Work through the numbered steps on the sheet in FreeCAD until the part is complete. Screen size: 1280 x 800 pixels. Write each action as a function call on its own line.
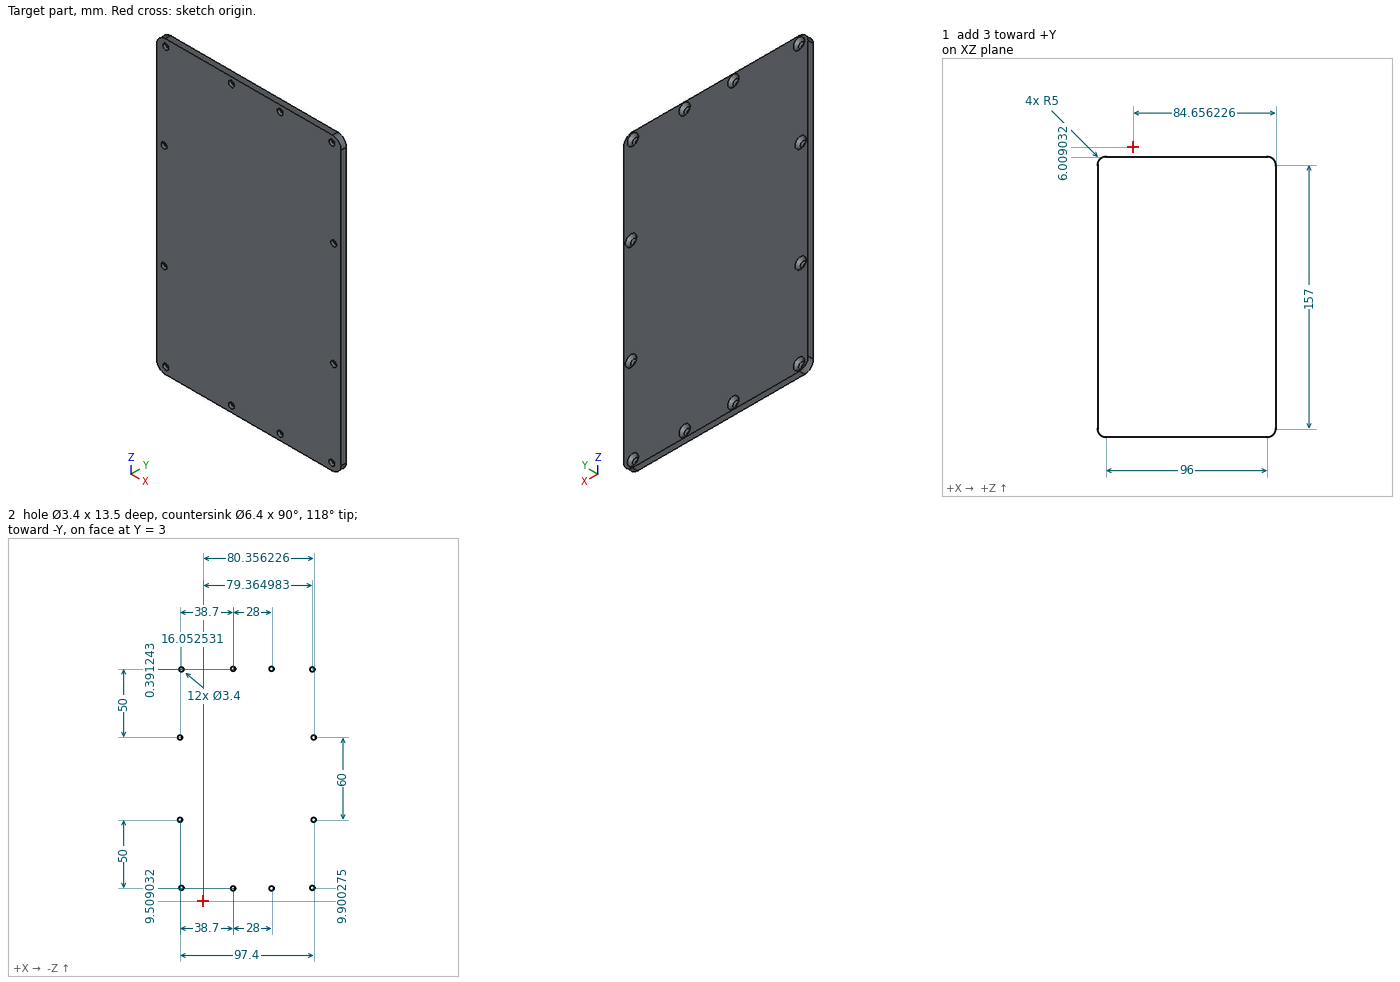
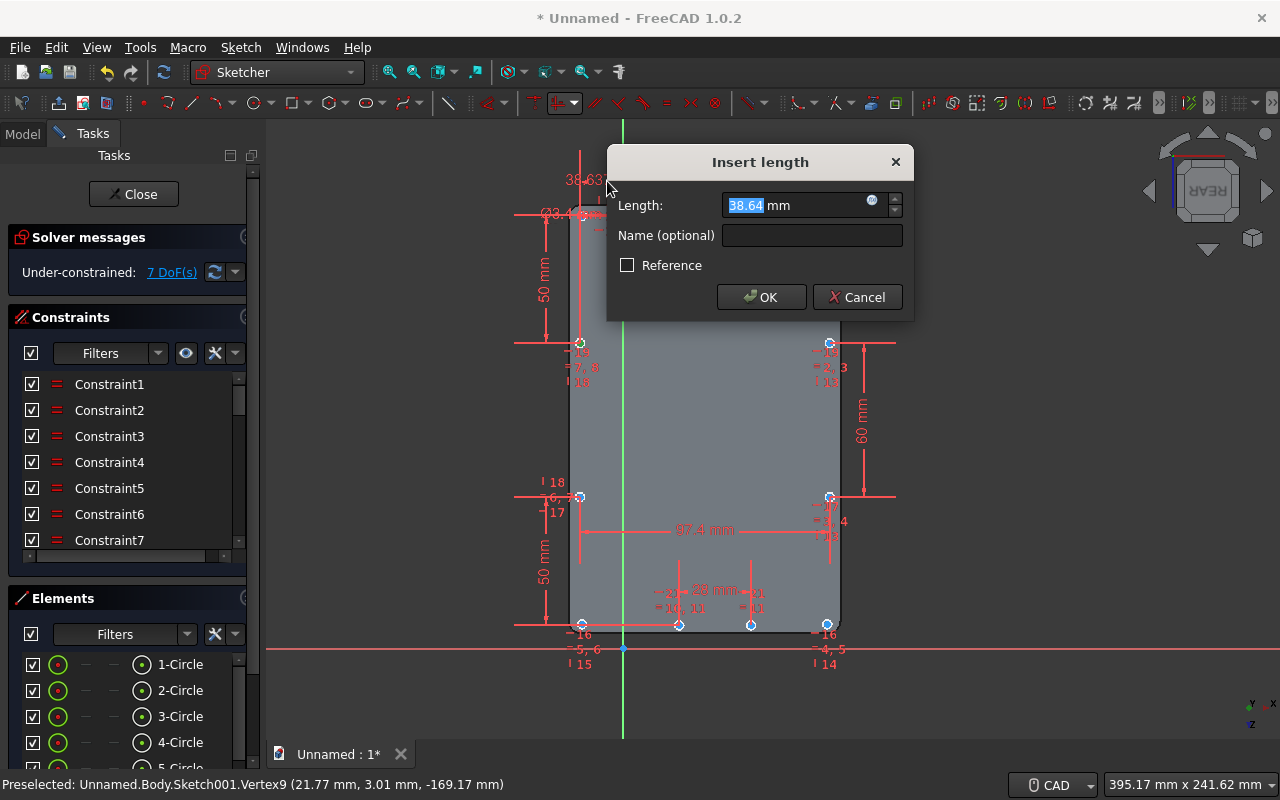
text(38.7)
key(Return)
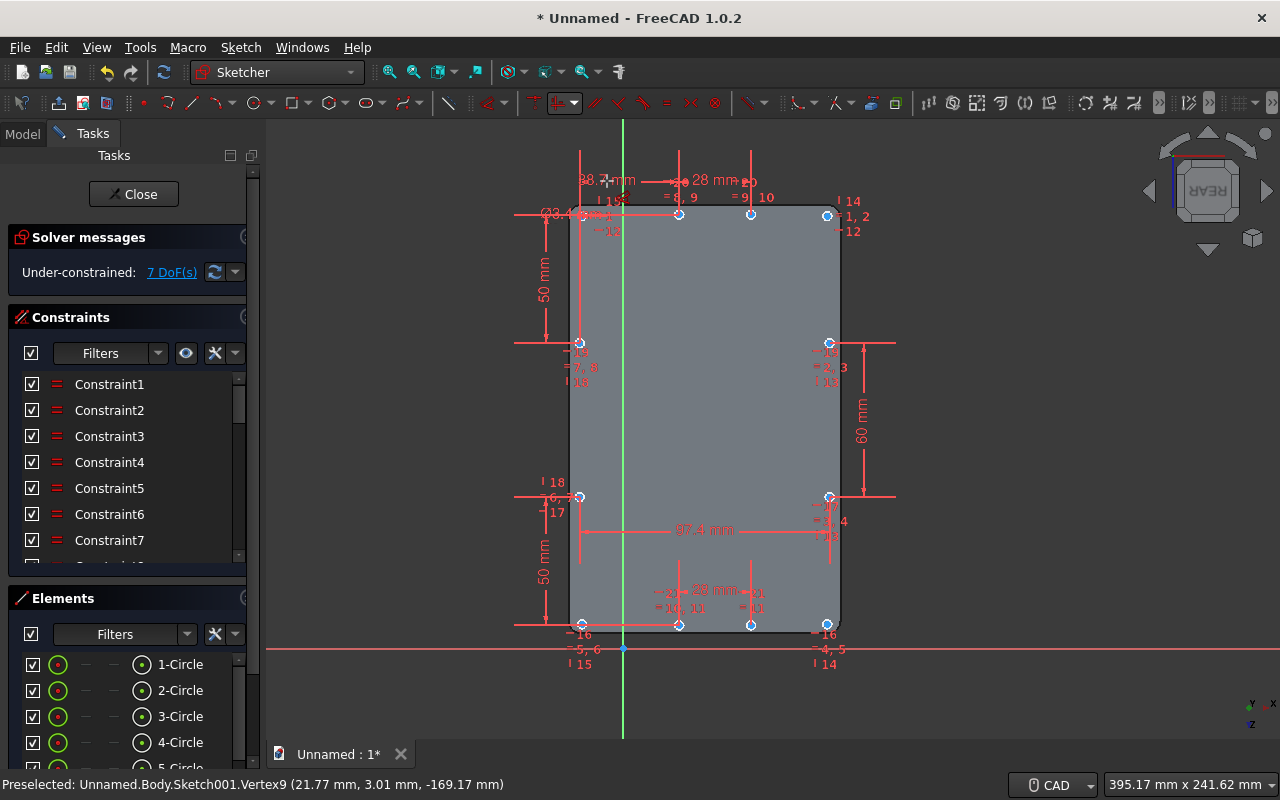
click(580, 497)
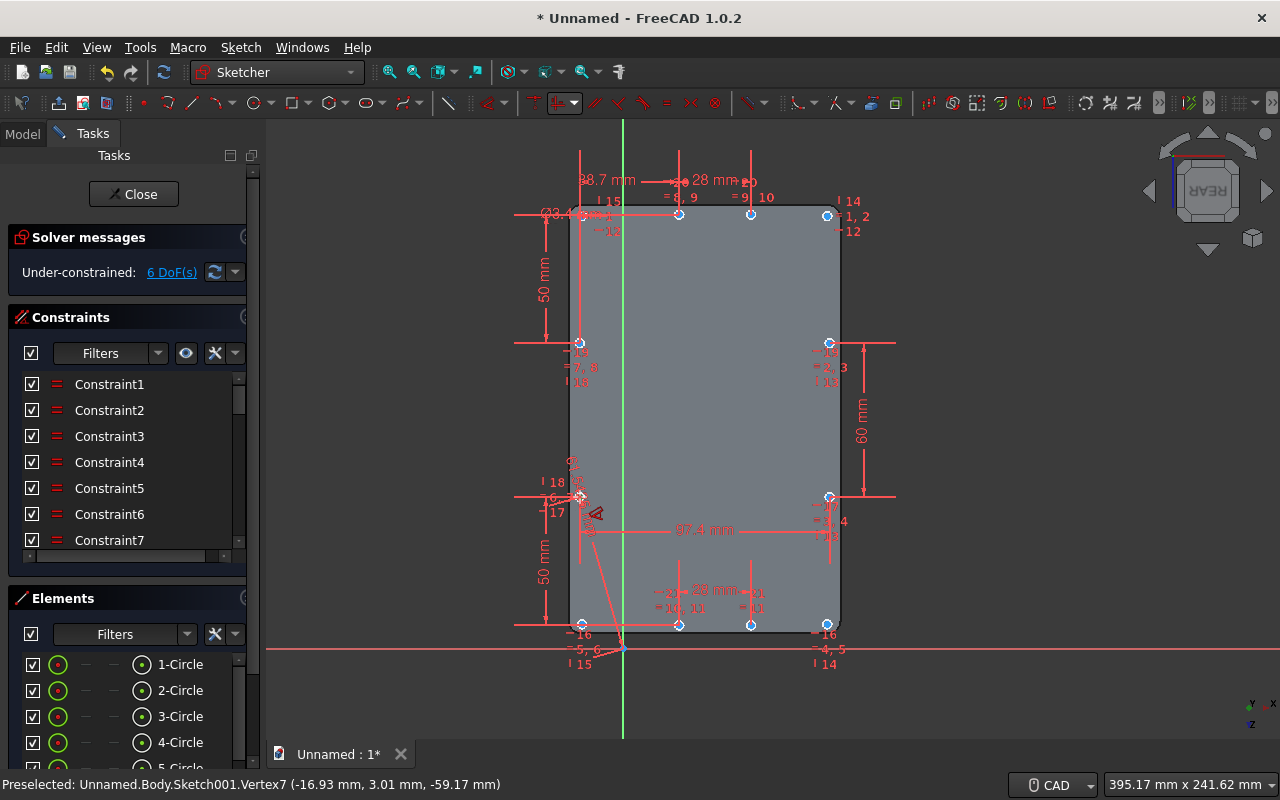
click(679, 625)
click(607, 463)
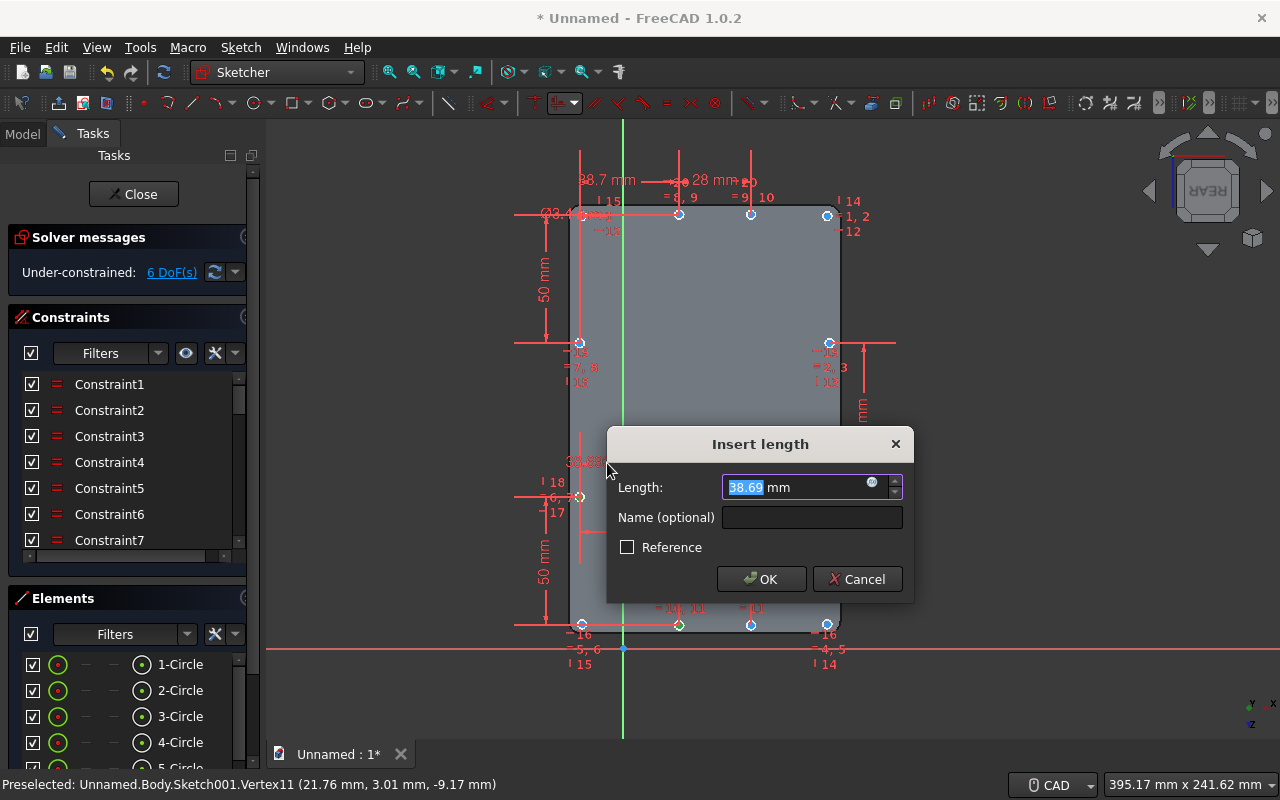
text(38.7)
key(Return)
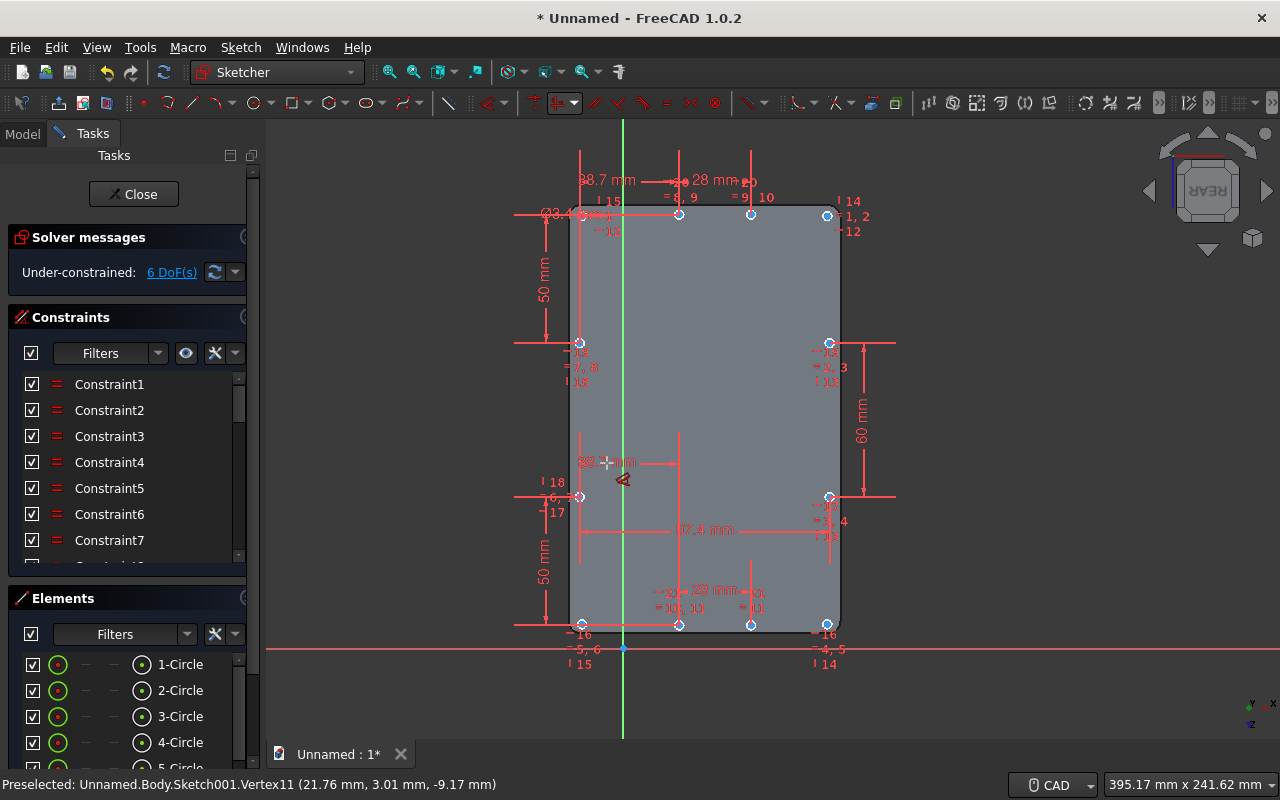
scroll(827, 624, up, 3)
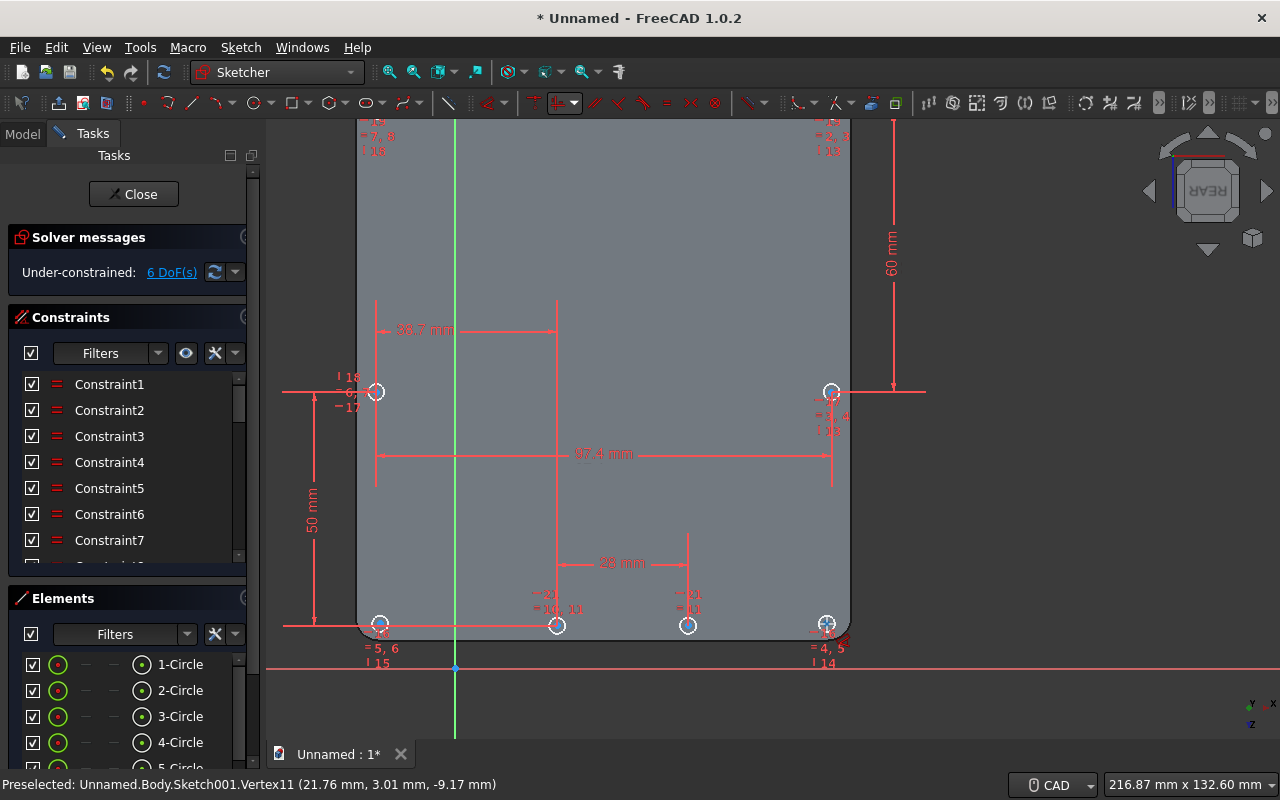
click(827, 624)
click(861, 646)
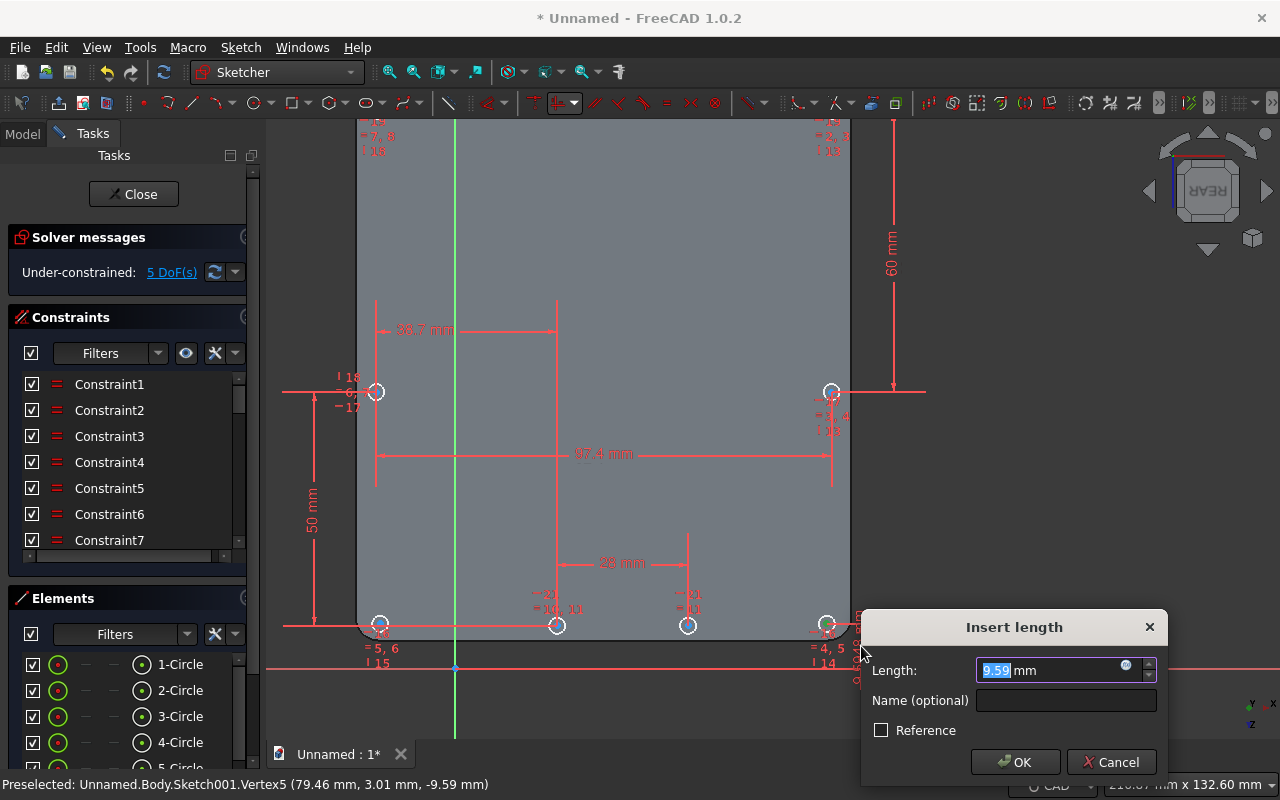
text(9.900275)
key(Return)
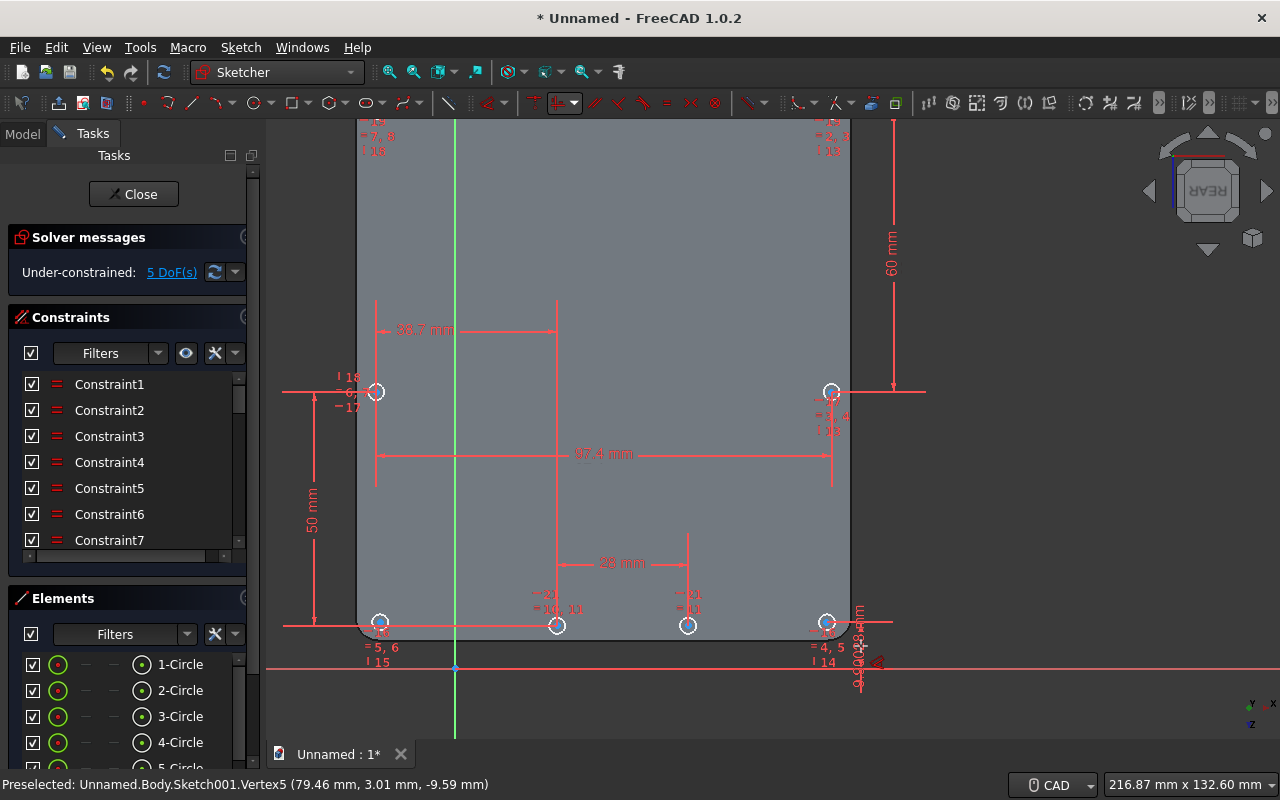
click(557, 626)
click(421, 647)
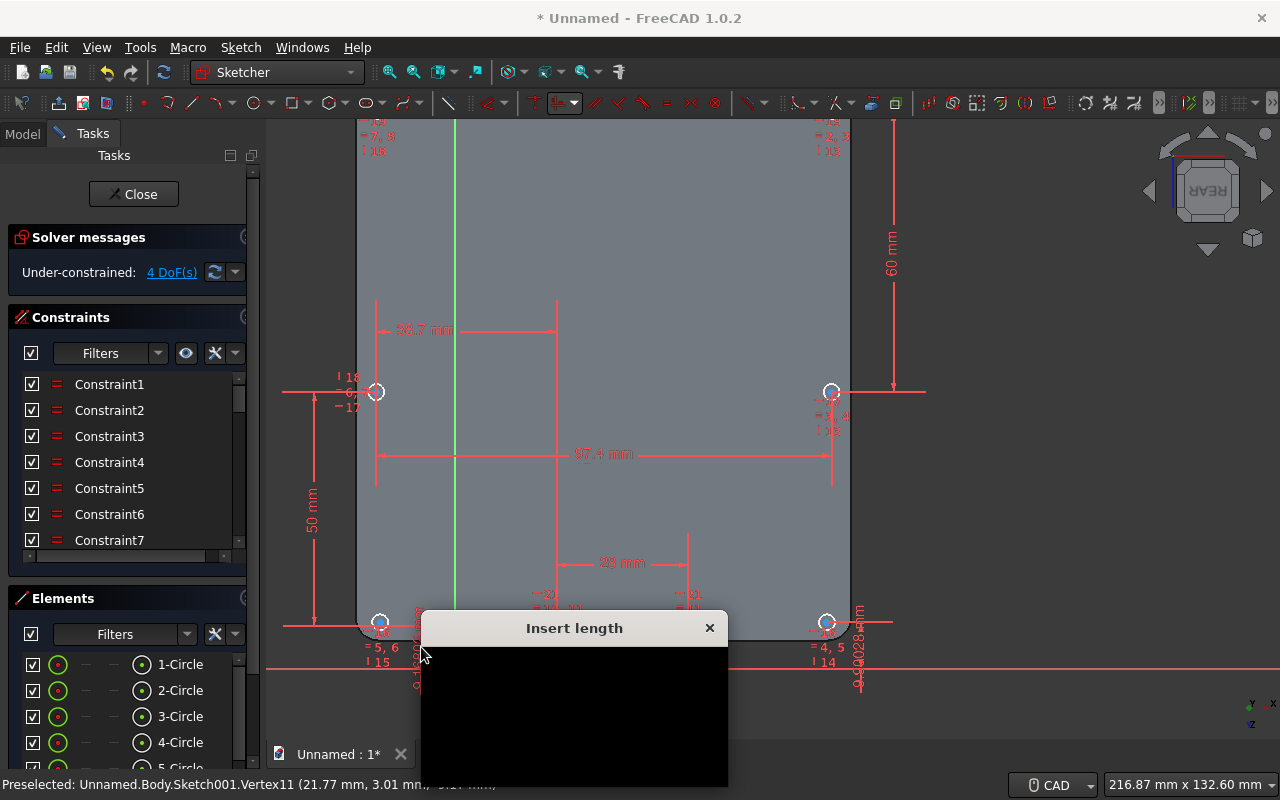
text(9.509032)
key(Return)